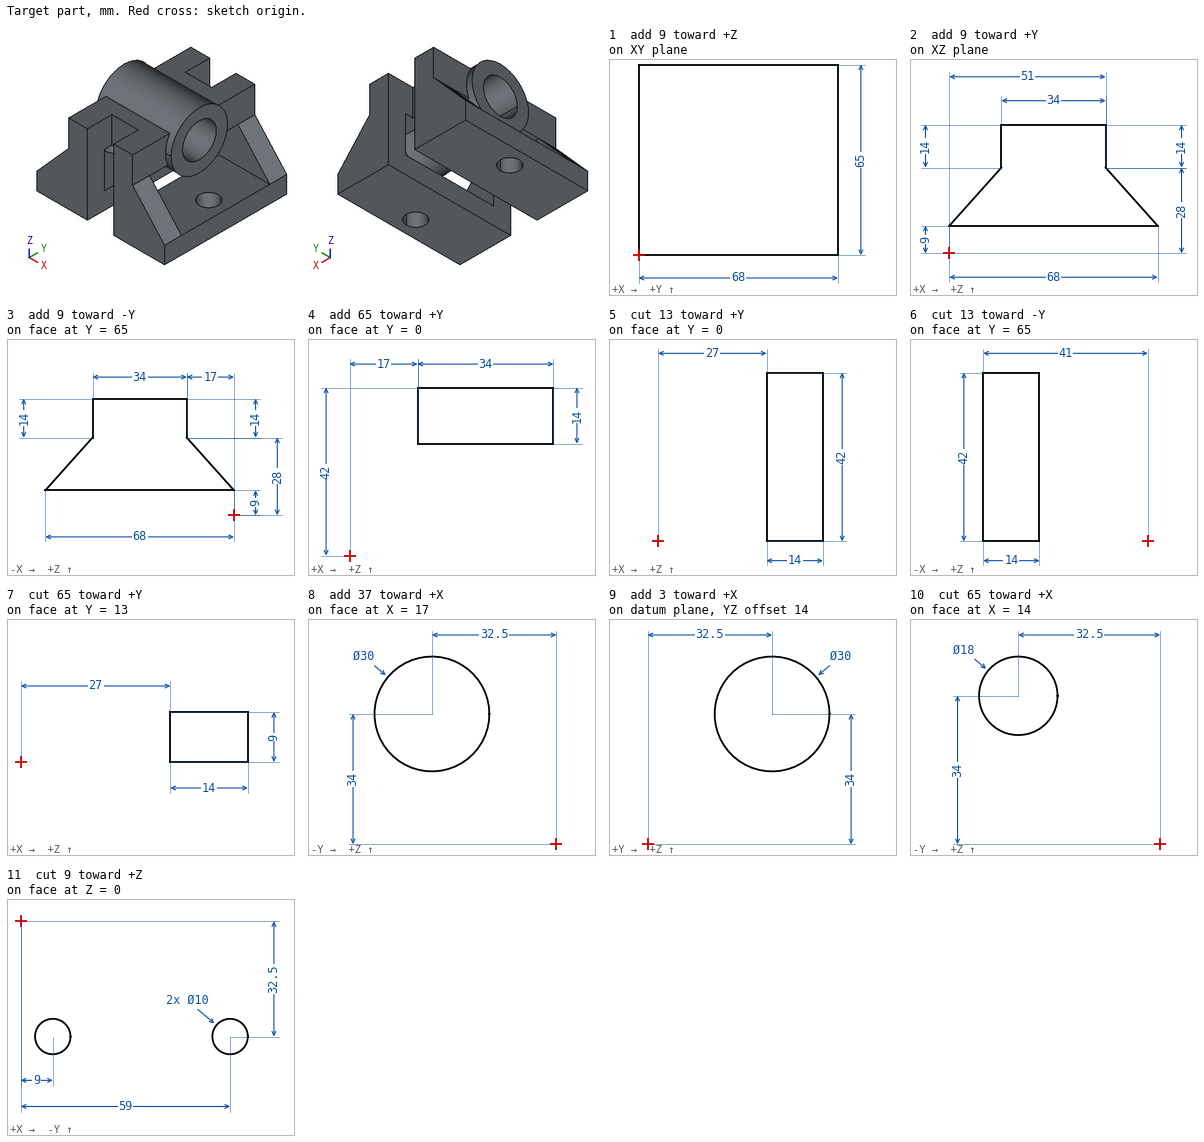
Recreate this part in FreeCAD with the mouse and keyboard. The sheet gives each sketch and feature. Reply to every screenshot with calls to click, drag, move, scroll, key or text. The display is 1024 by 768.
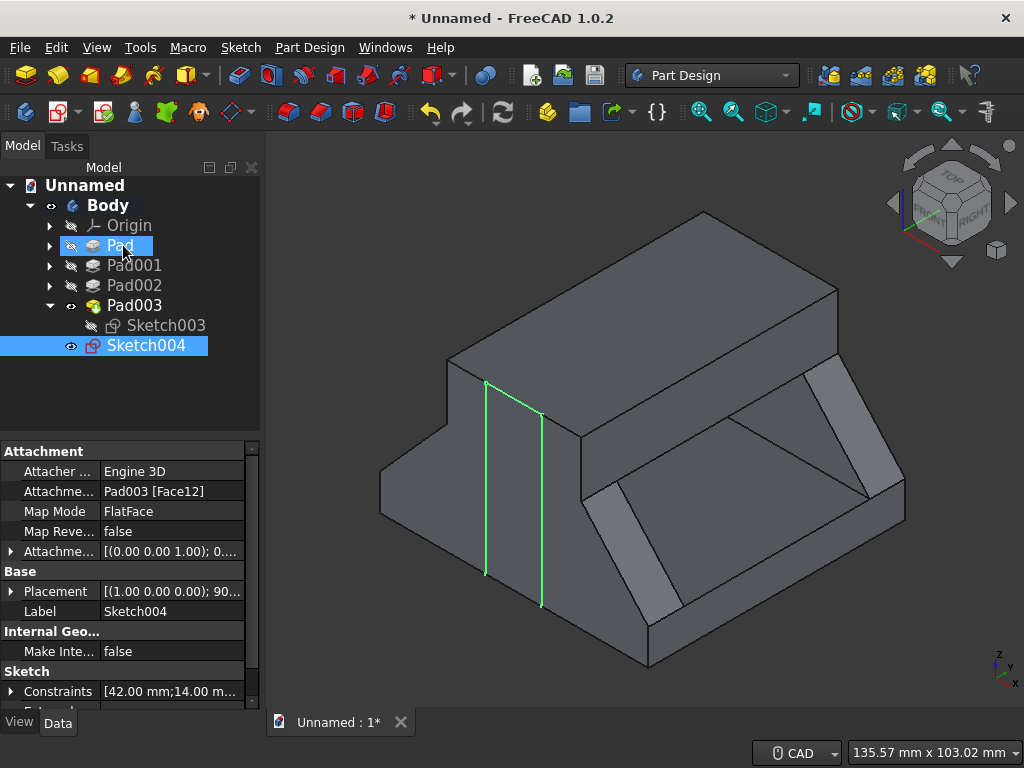
click(240, 76)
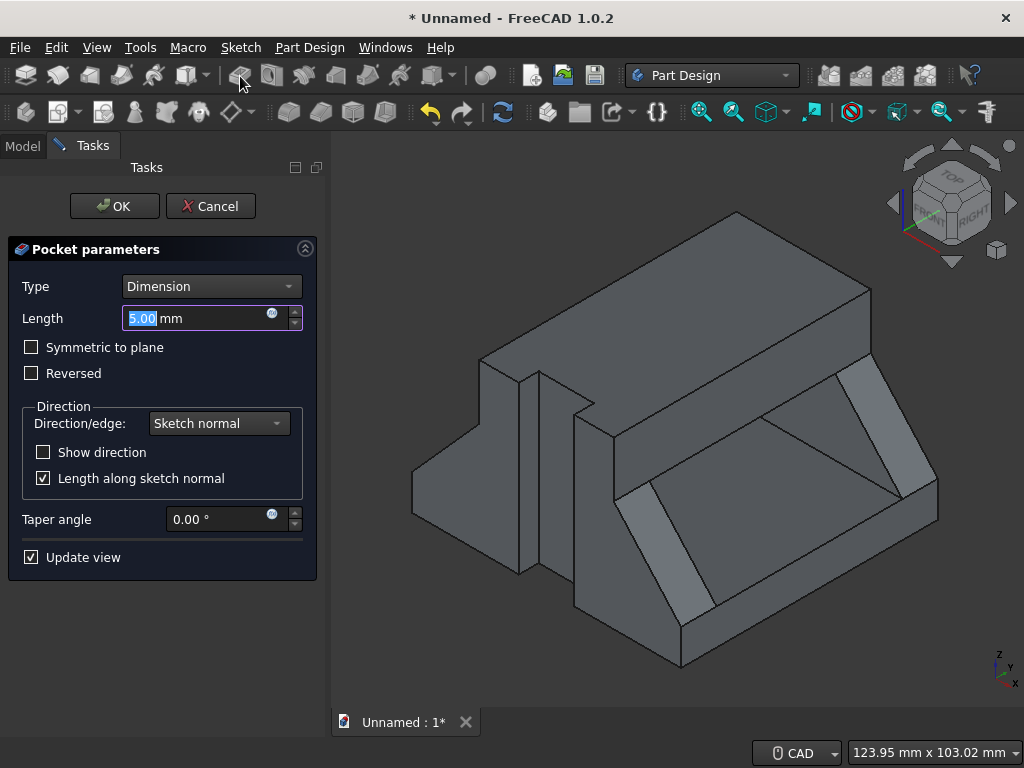
text(13)
key(Tab)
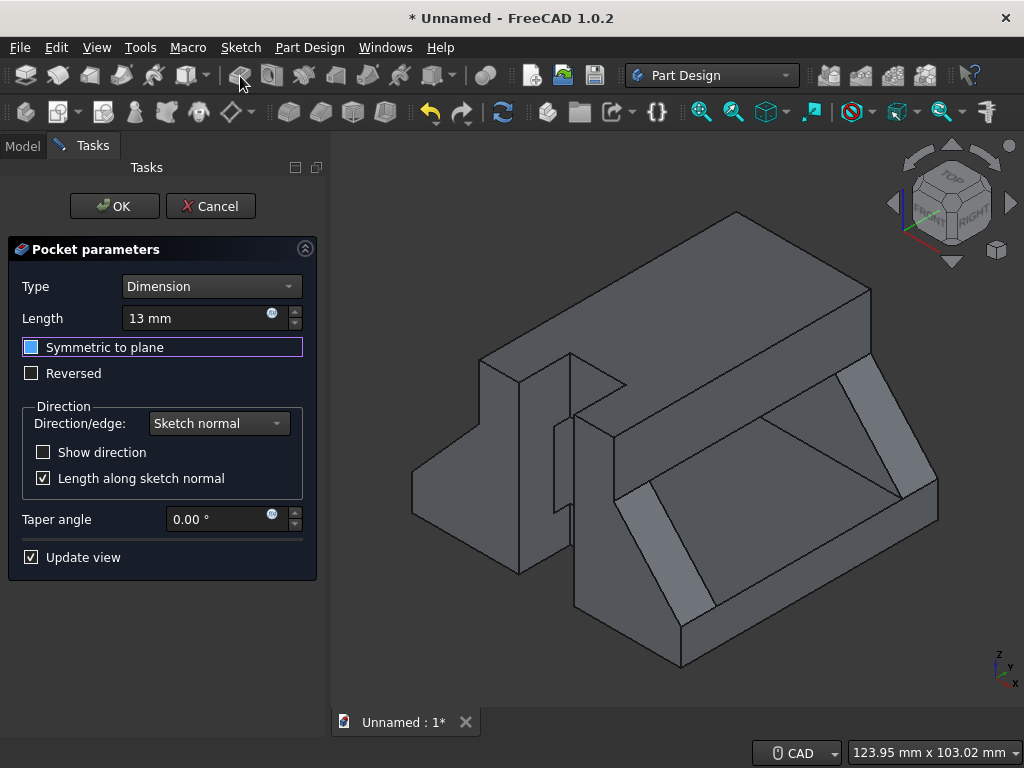
click(115, 206)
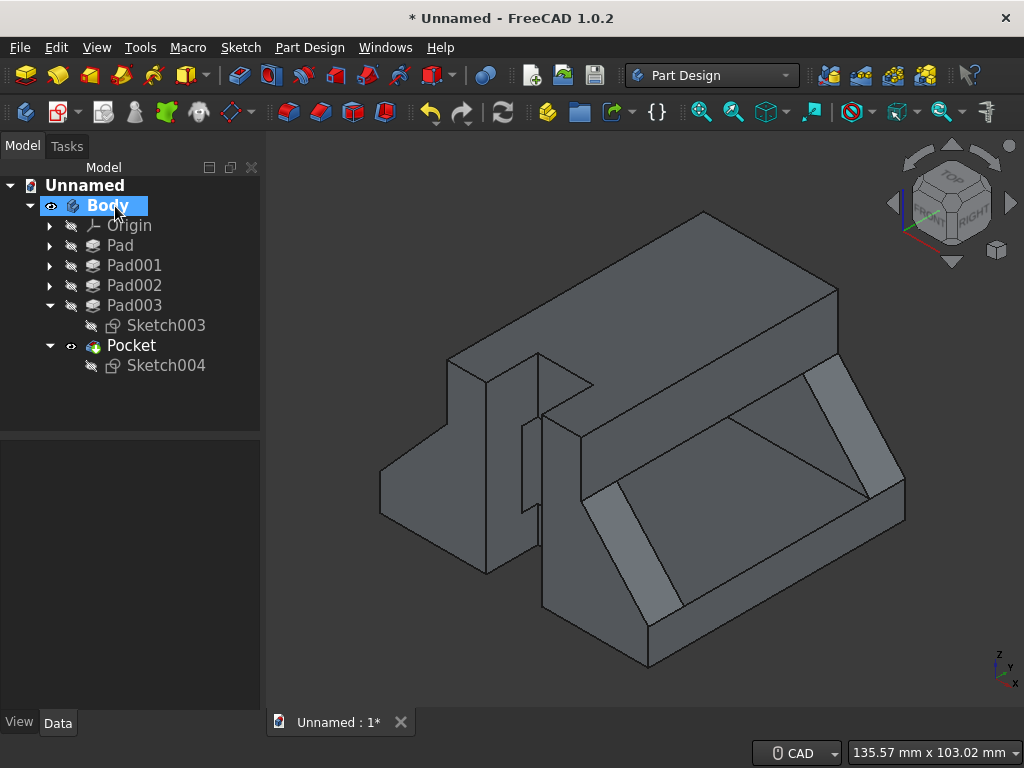
key(4)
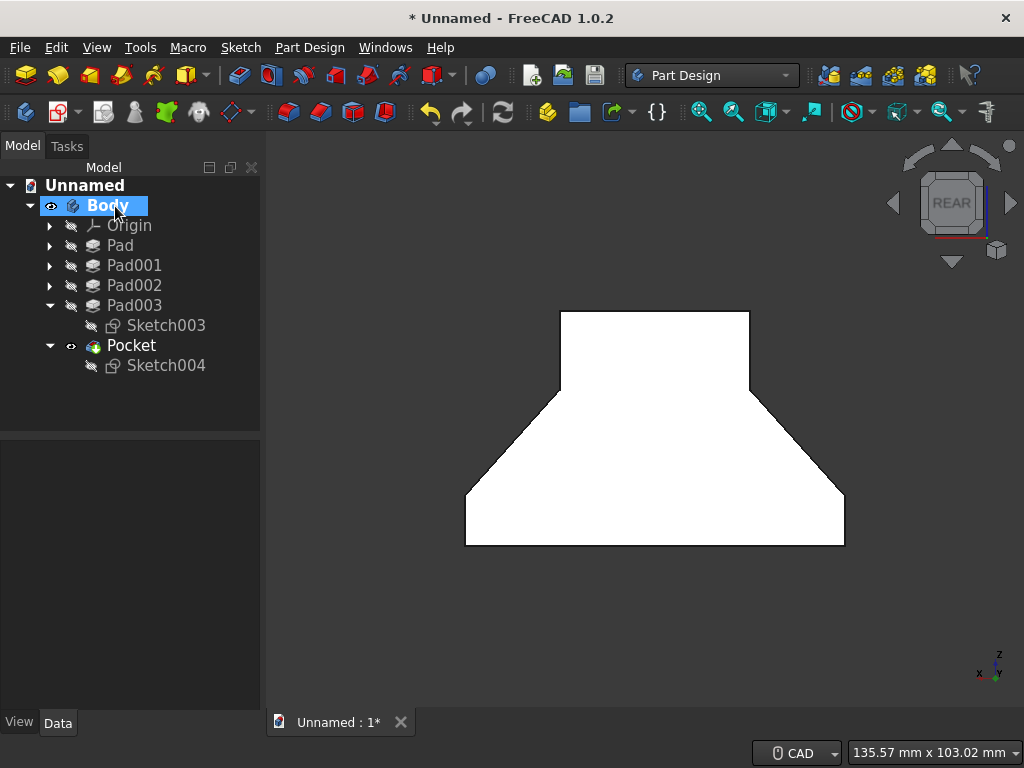
click(655, 428)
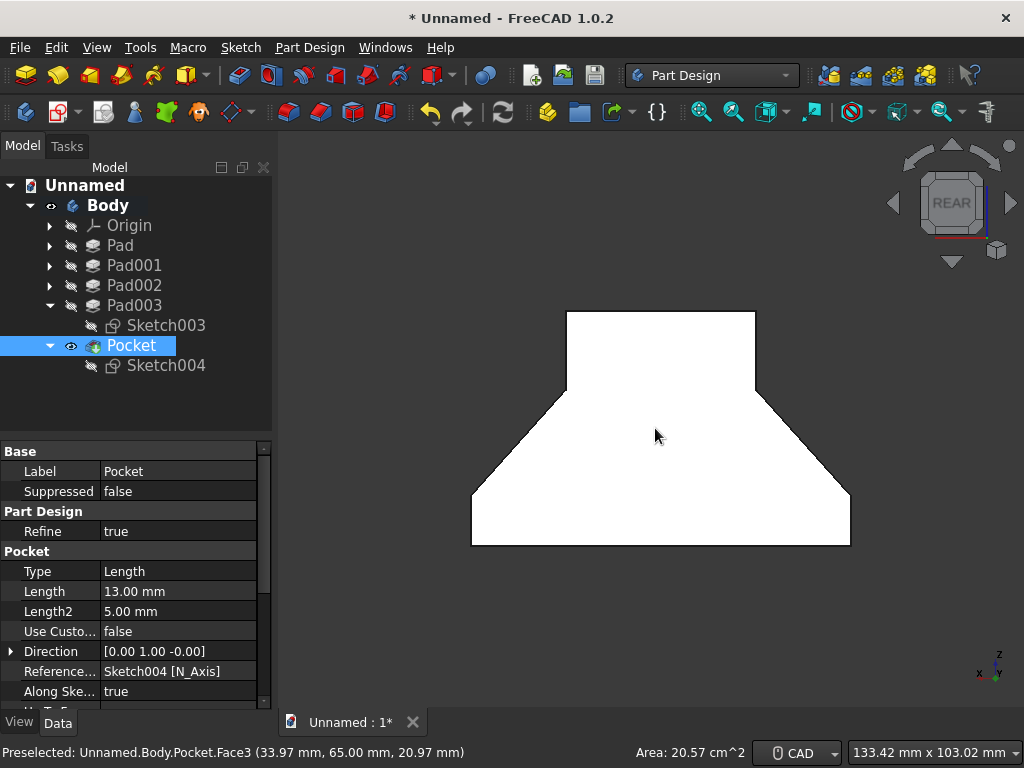
click(58, 112)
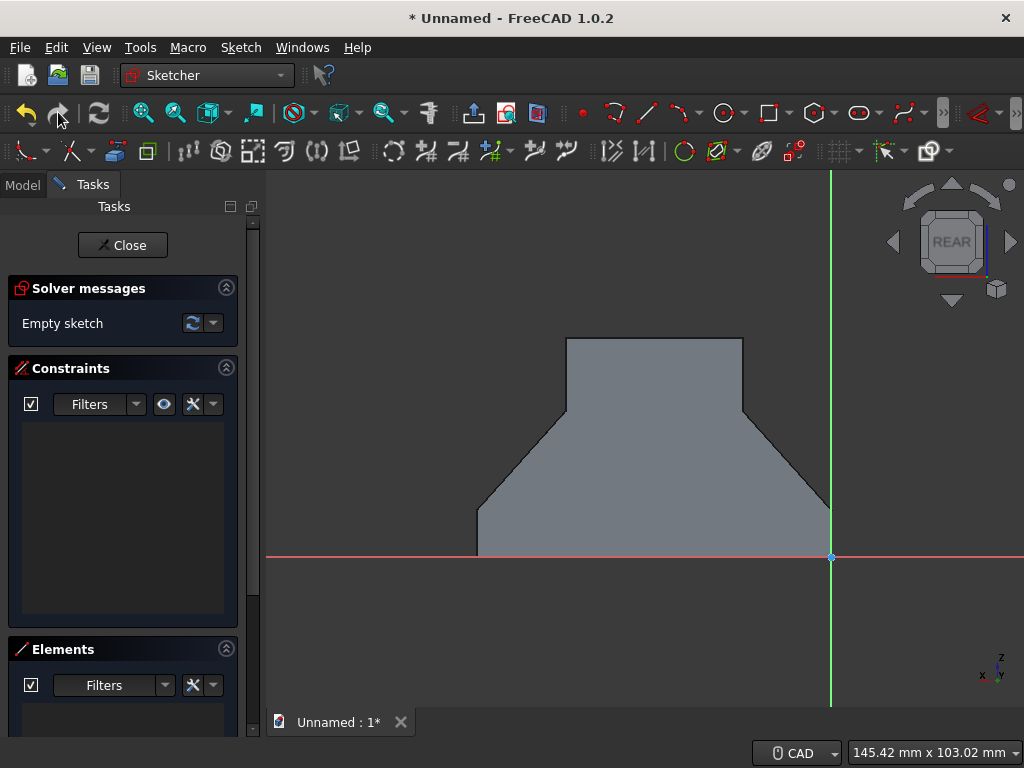
scroll(859, 466, up, 2)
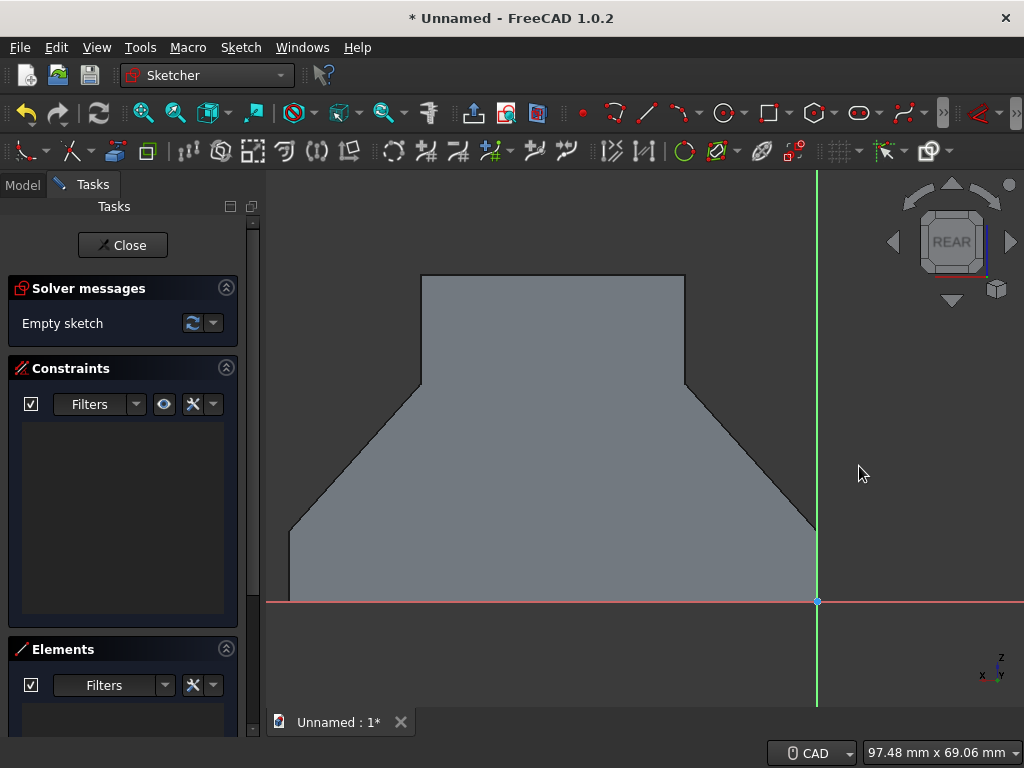
click(770, 114)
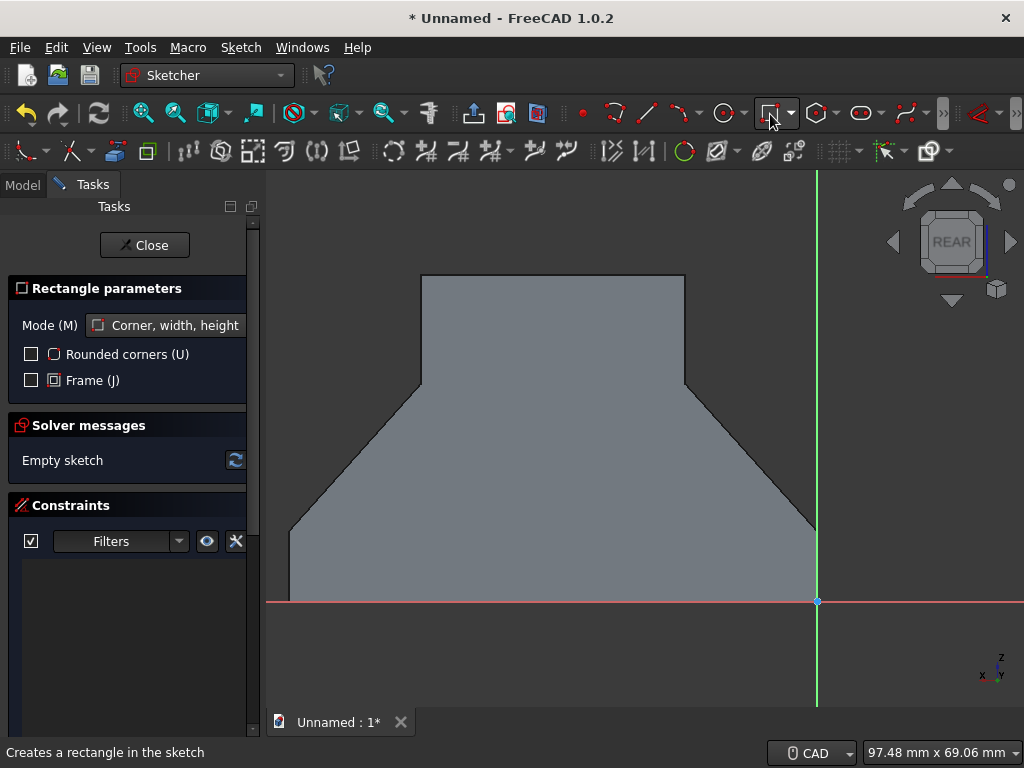
click(499, 275)
click(607, 602)
key(Escape)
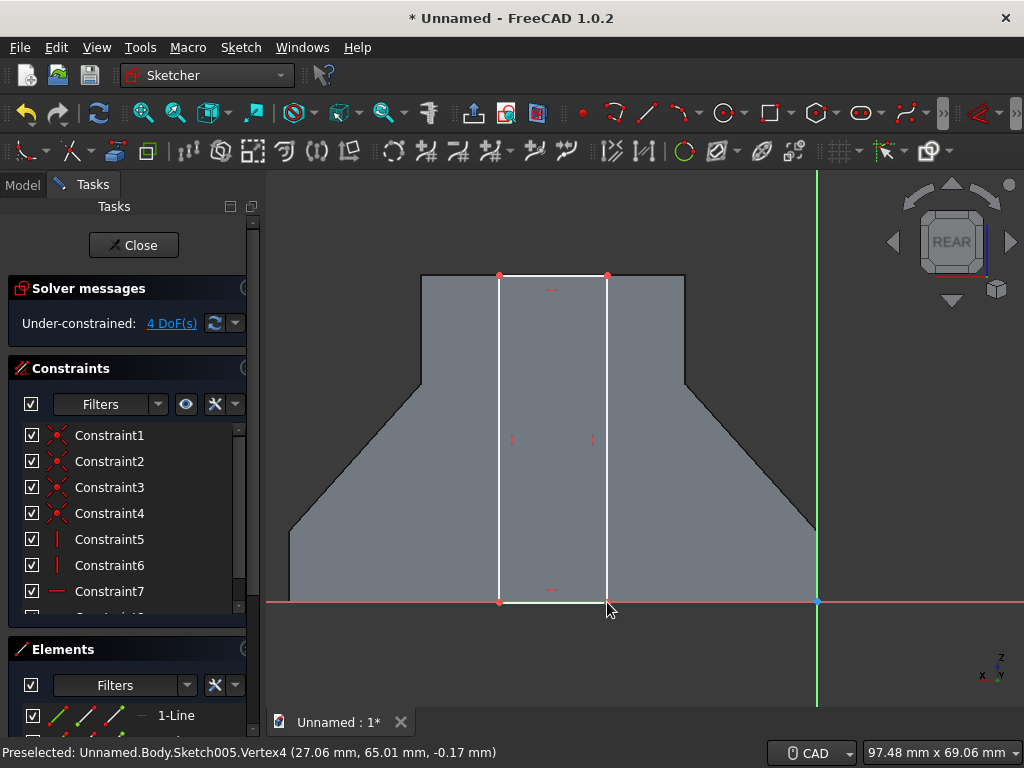
click(499, 603)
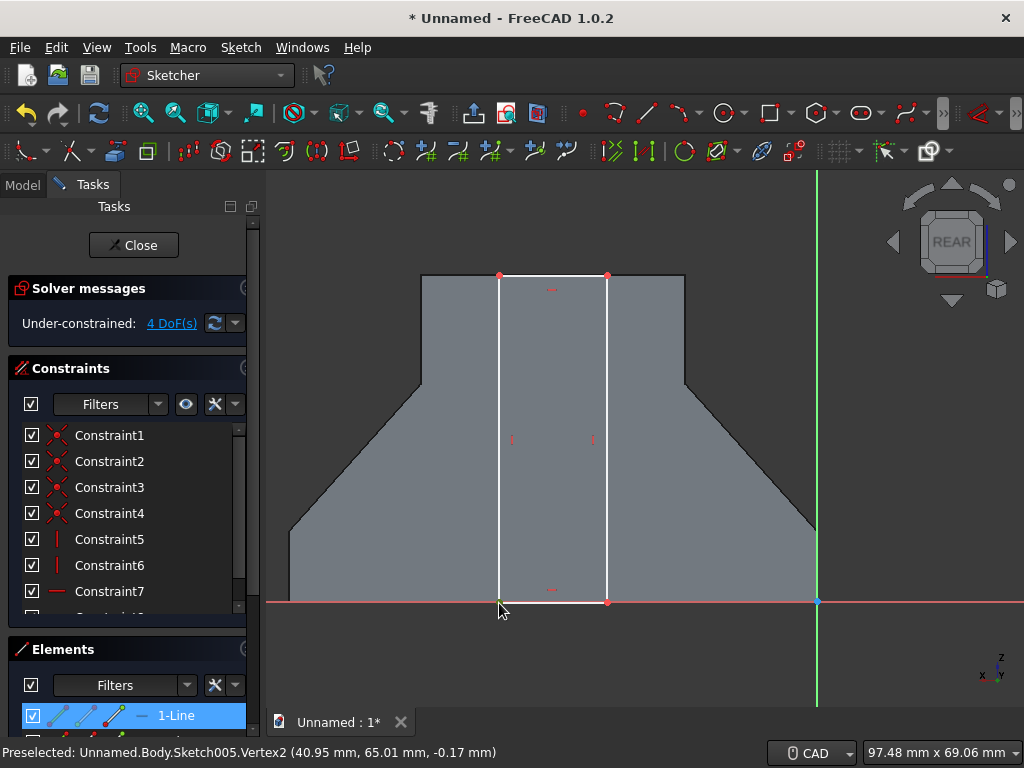
click(334, 602)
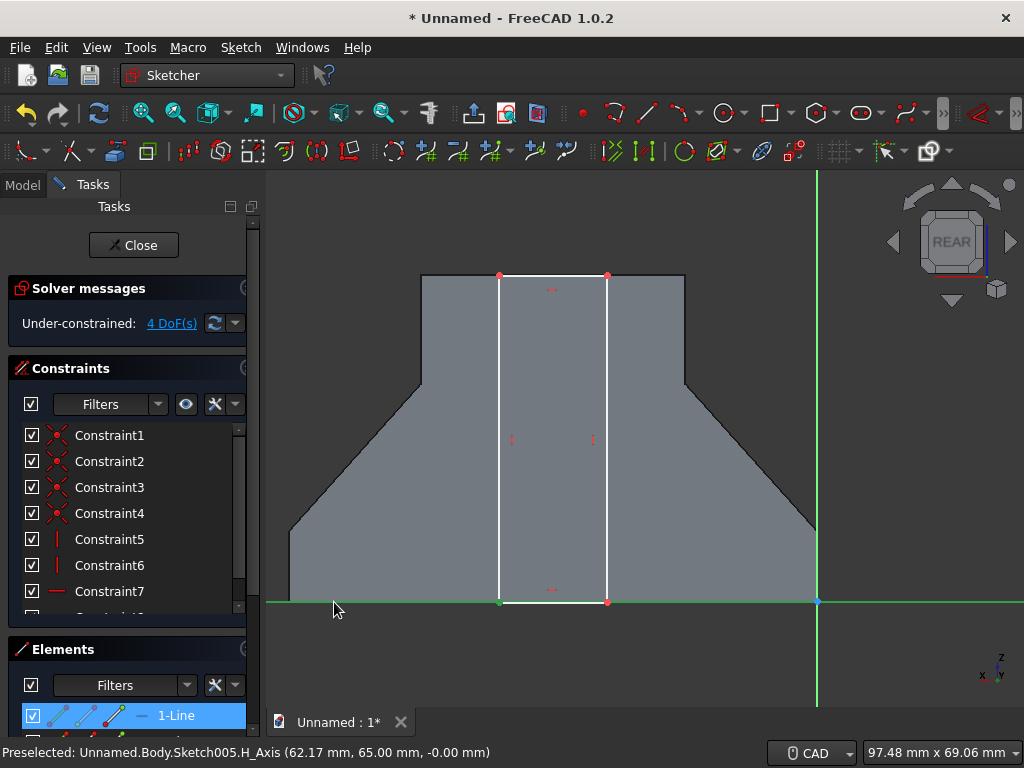
key(c)